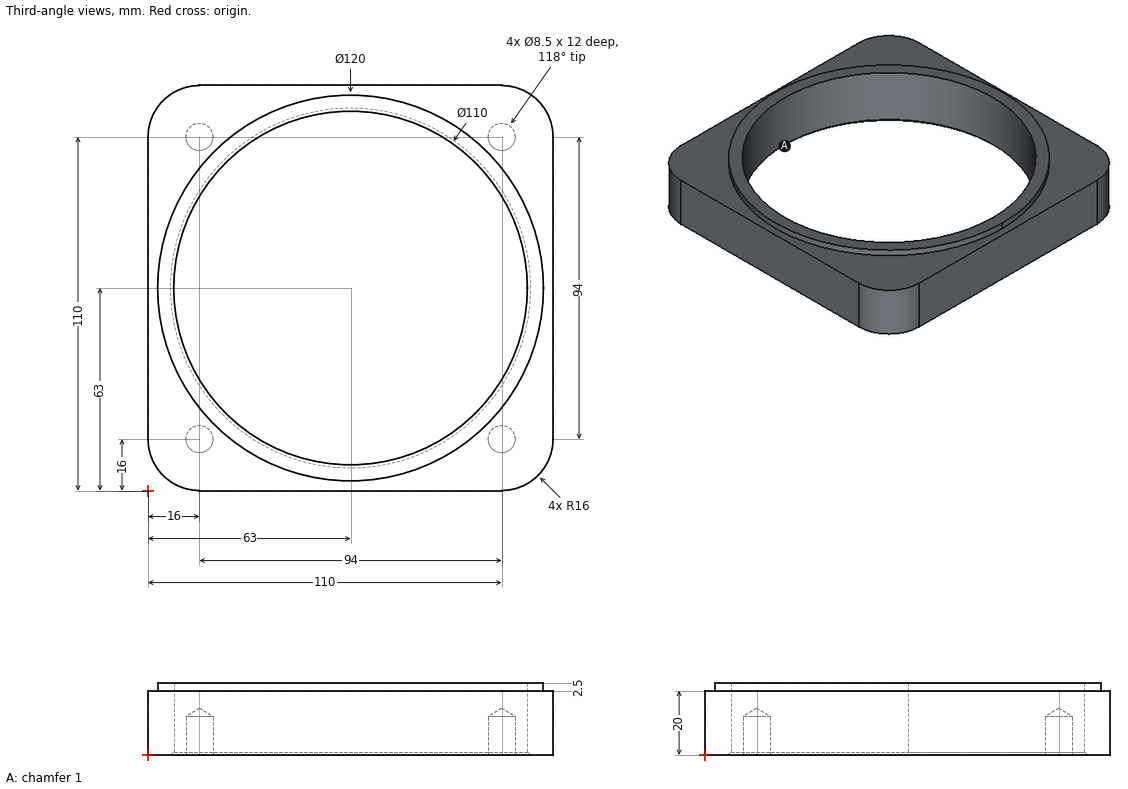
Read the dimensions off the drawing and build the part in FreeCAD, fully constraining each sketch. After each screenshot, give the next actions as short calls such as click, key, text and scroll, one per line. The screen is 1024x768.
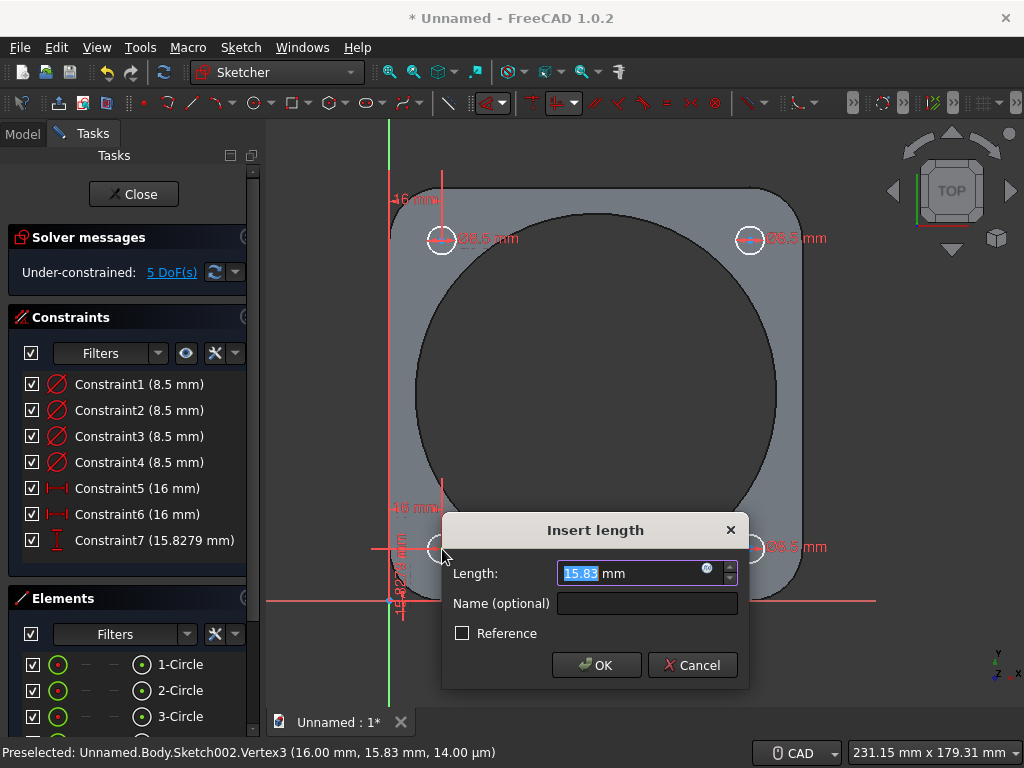
text(16)
key(Return)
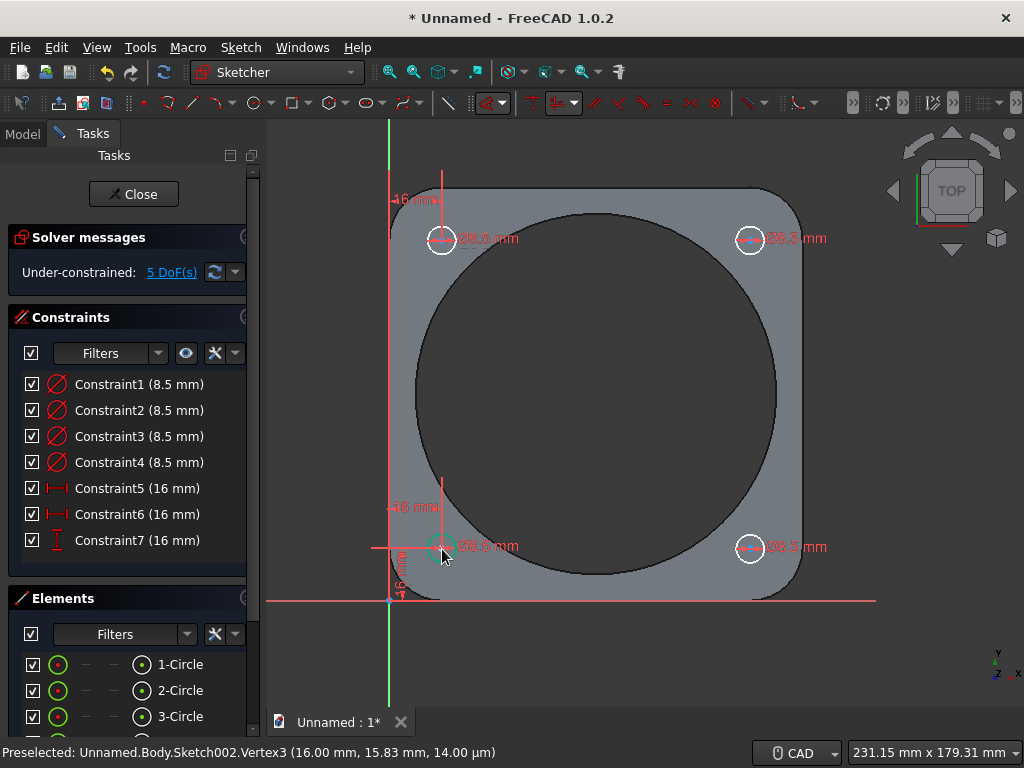
click(750, 549)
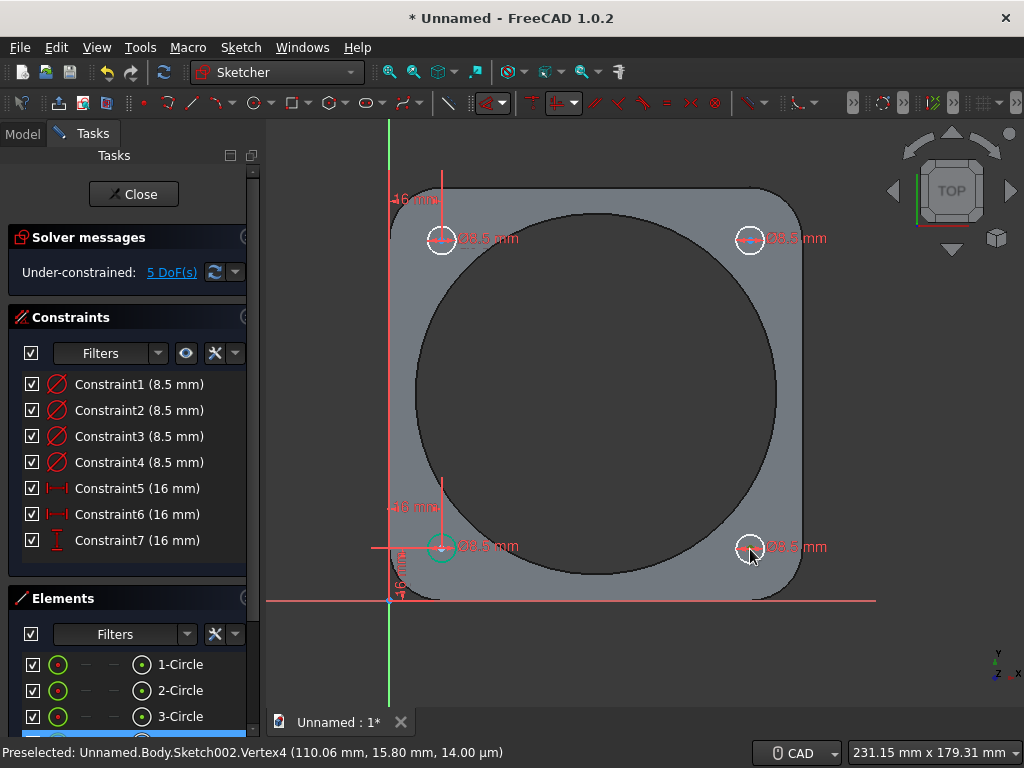
click(504, 104)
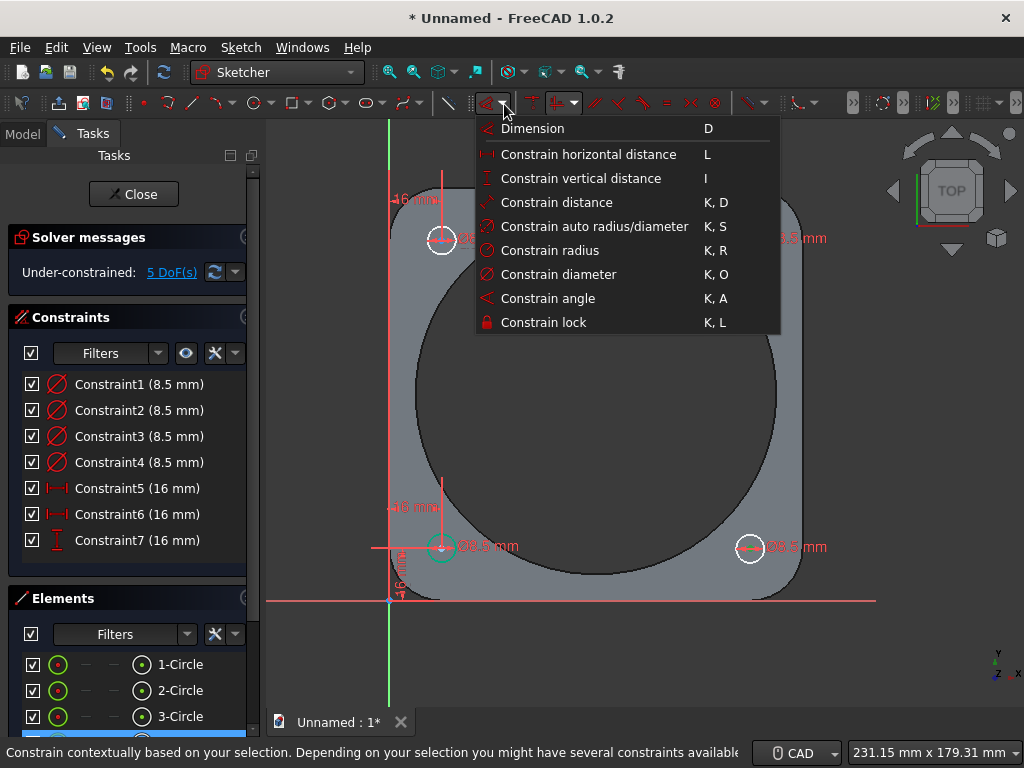
click(628, 178)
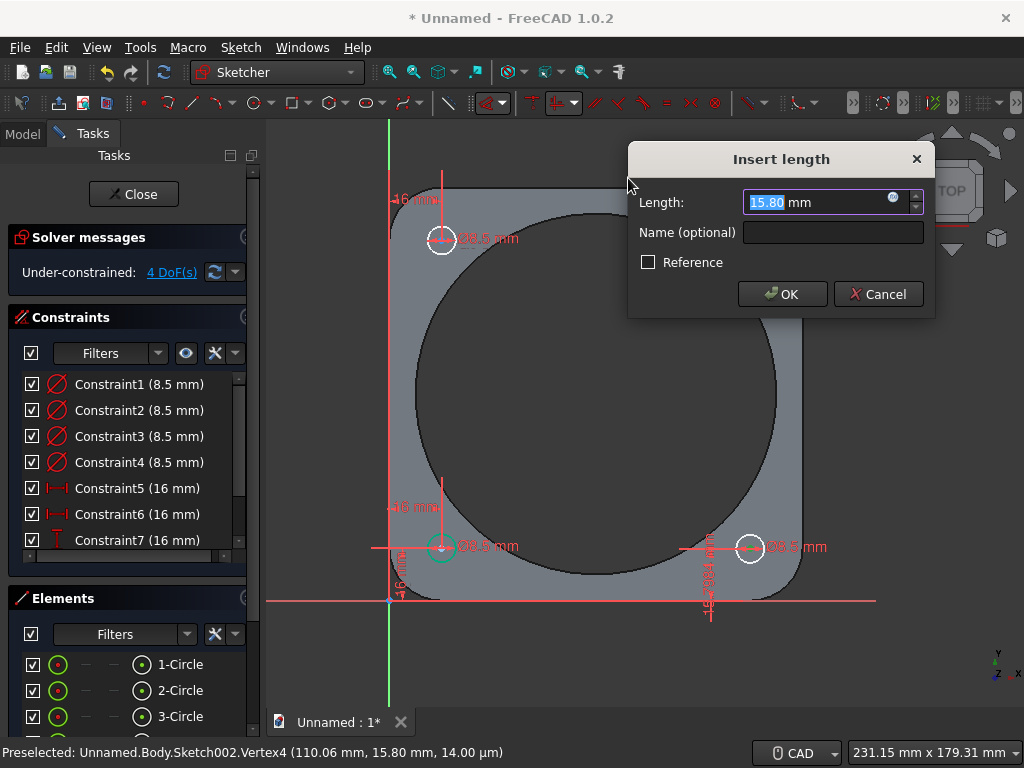
text(16)
key(Return)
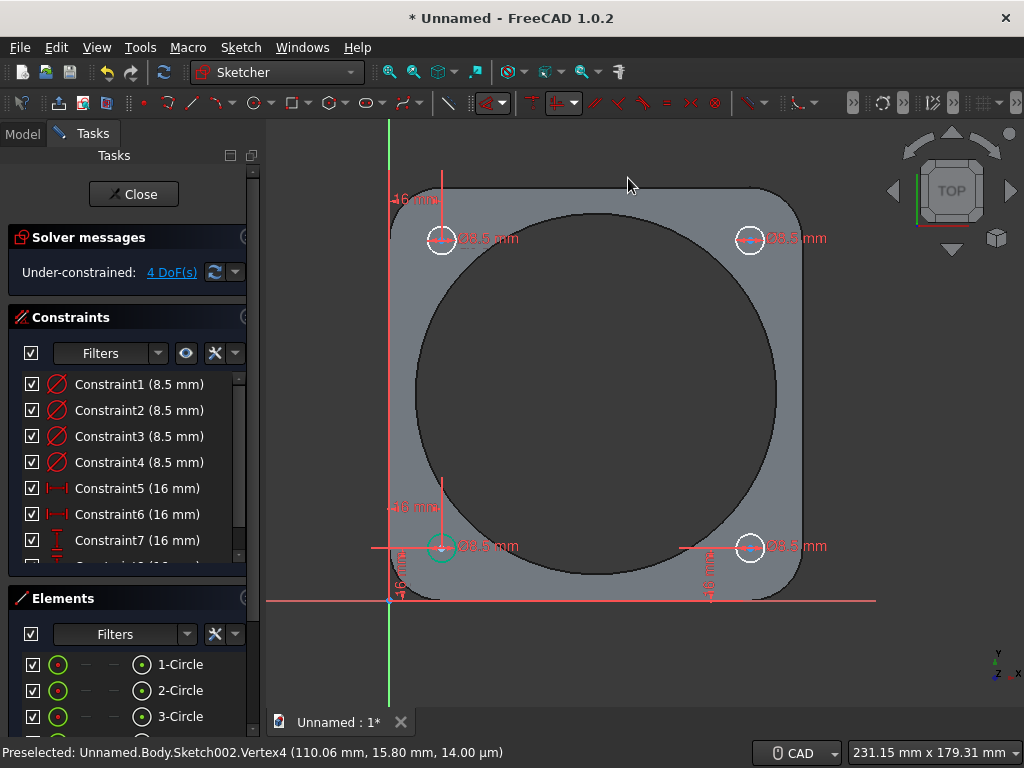
click(750, 240)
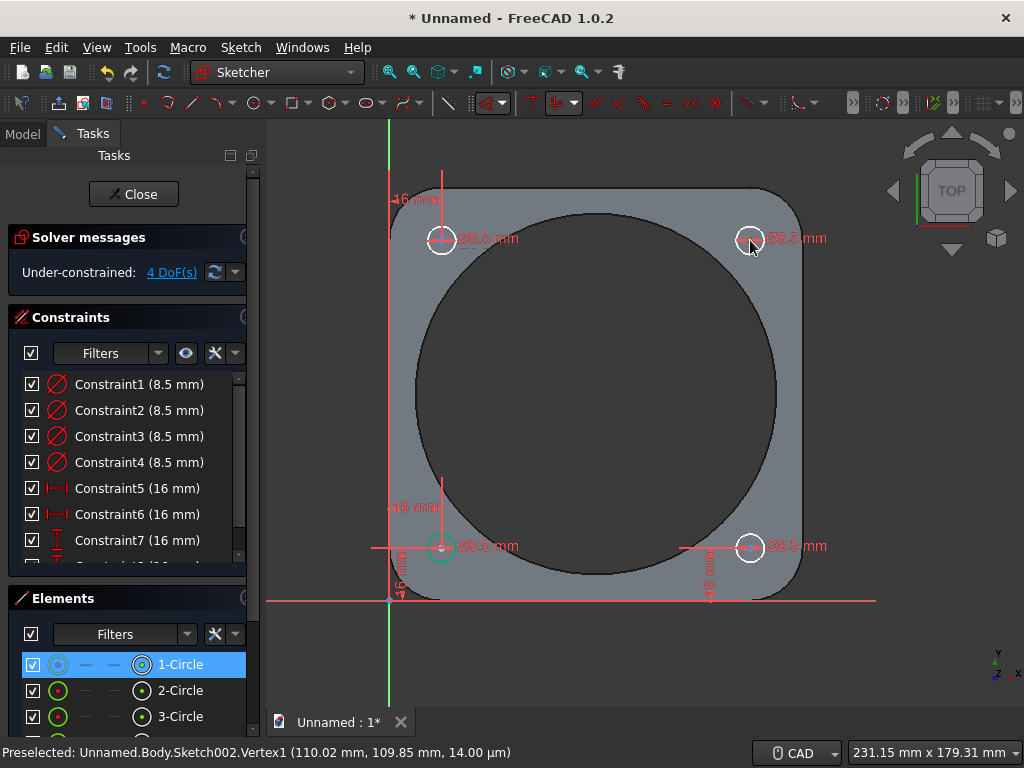
click(504, 104)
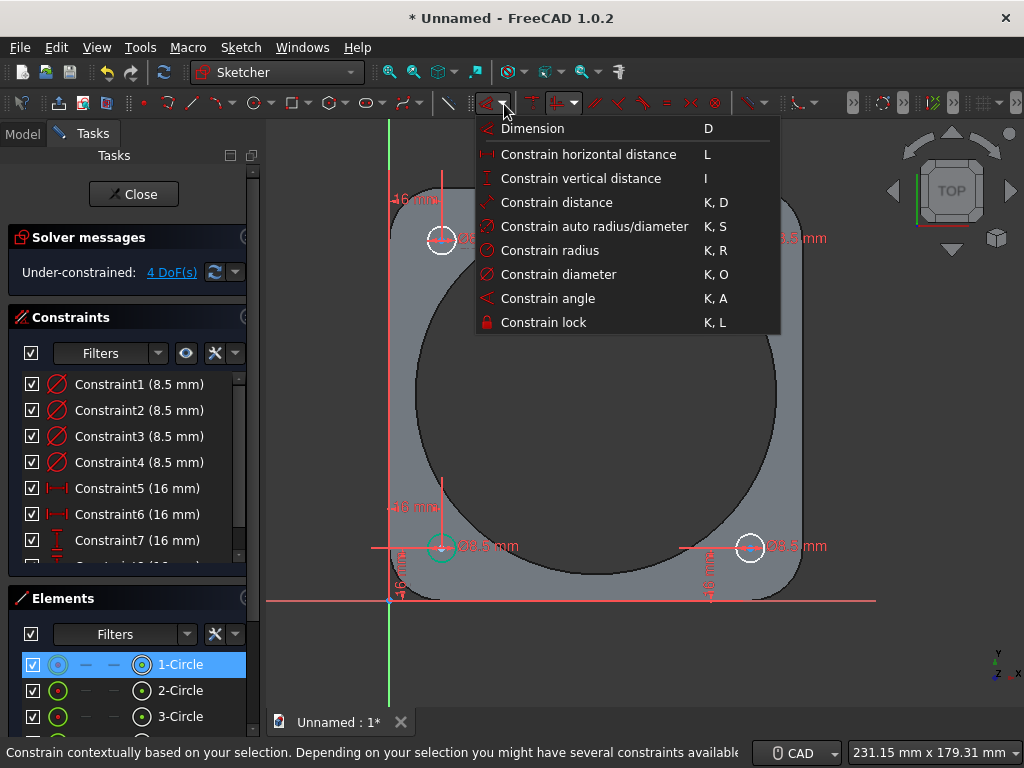
click(628, 154)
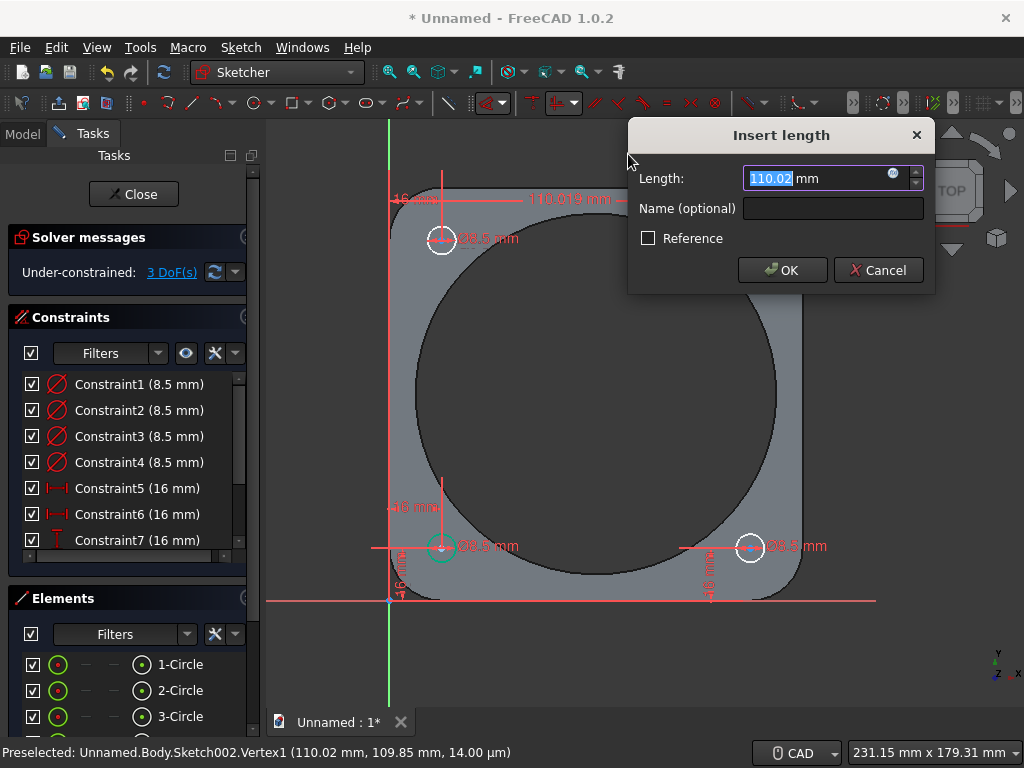
text(110)
key(Return)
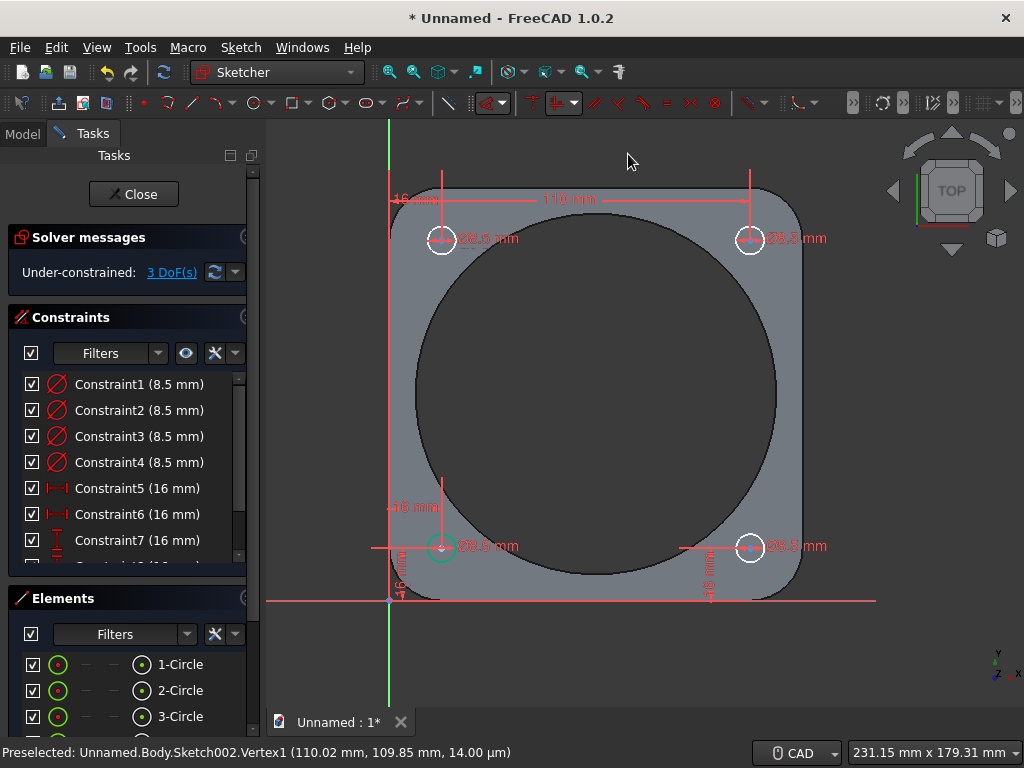
click(750, 240)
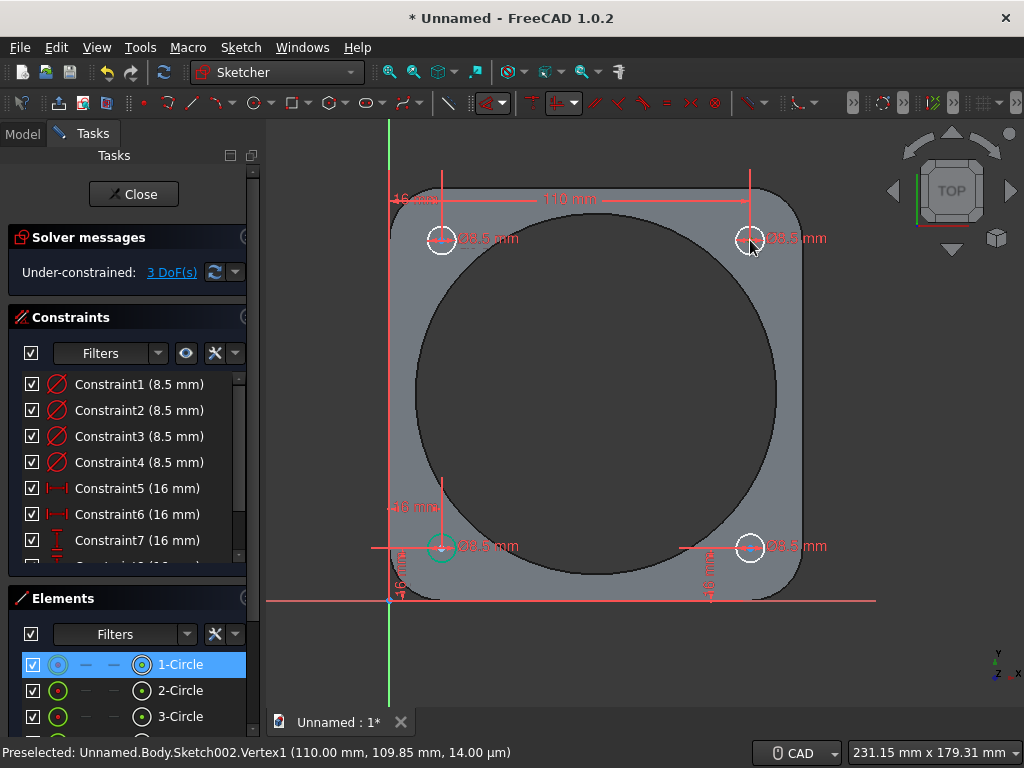
click(504, 104)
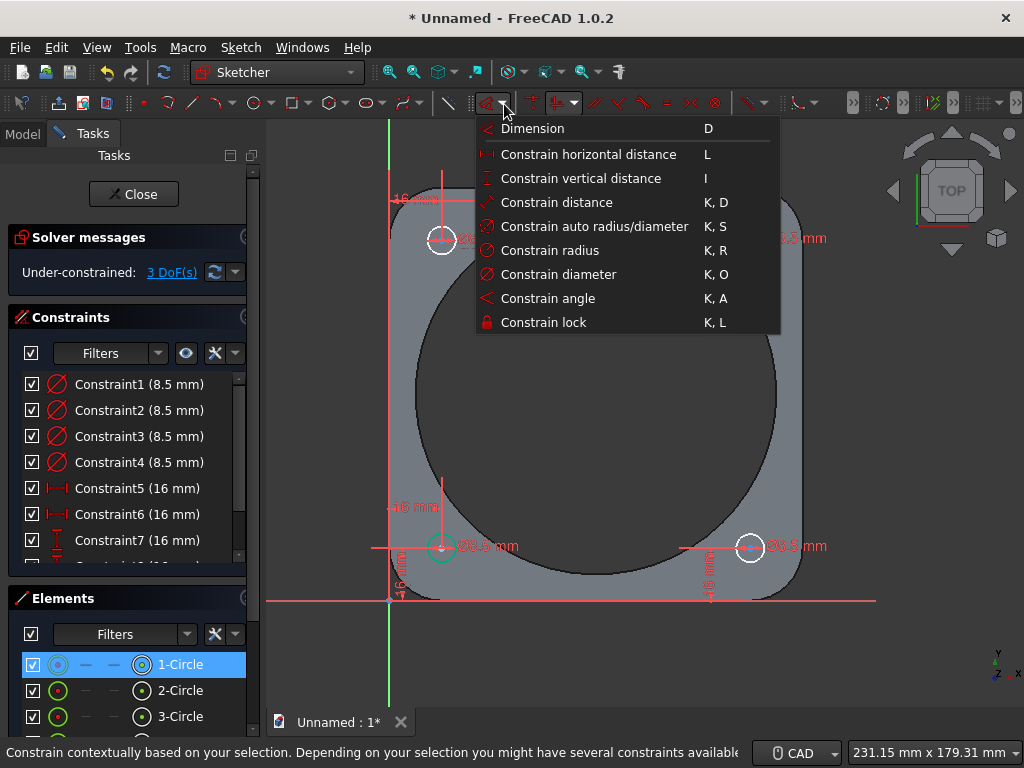
click(628, 178)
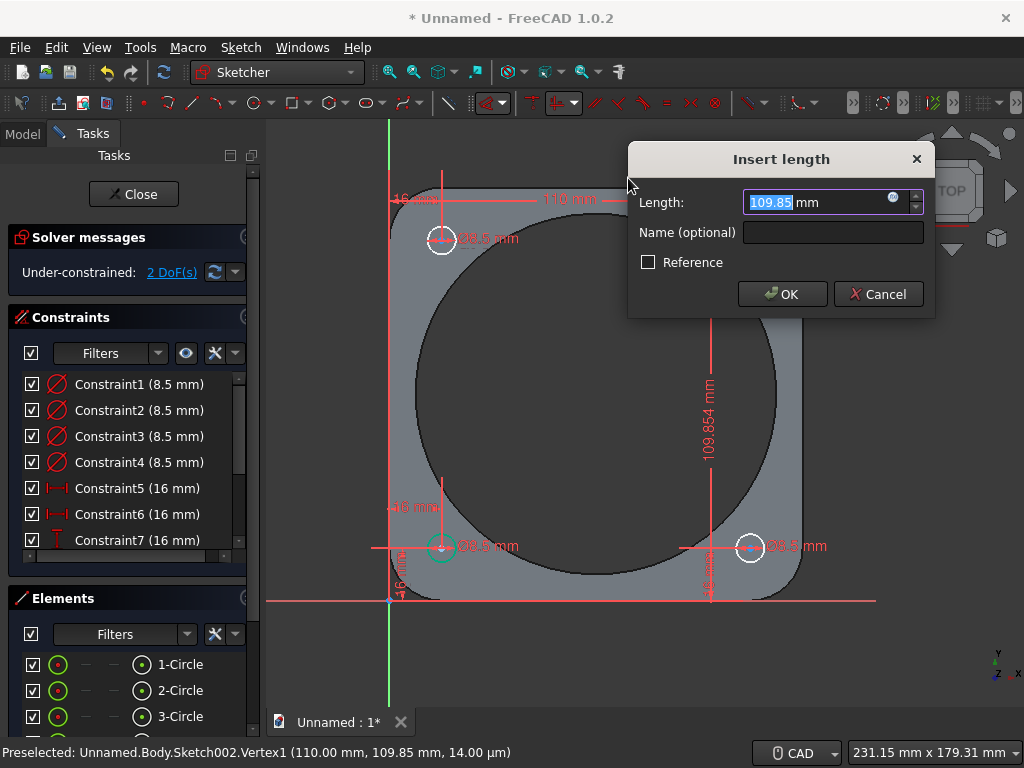
text(110)
key(Return)